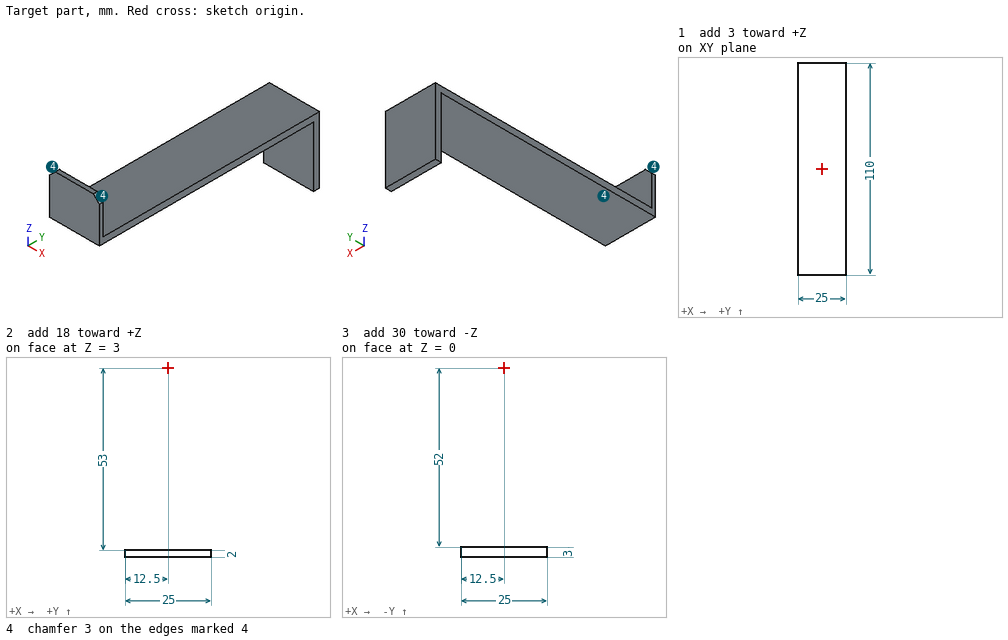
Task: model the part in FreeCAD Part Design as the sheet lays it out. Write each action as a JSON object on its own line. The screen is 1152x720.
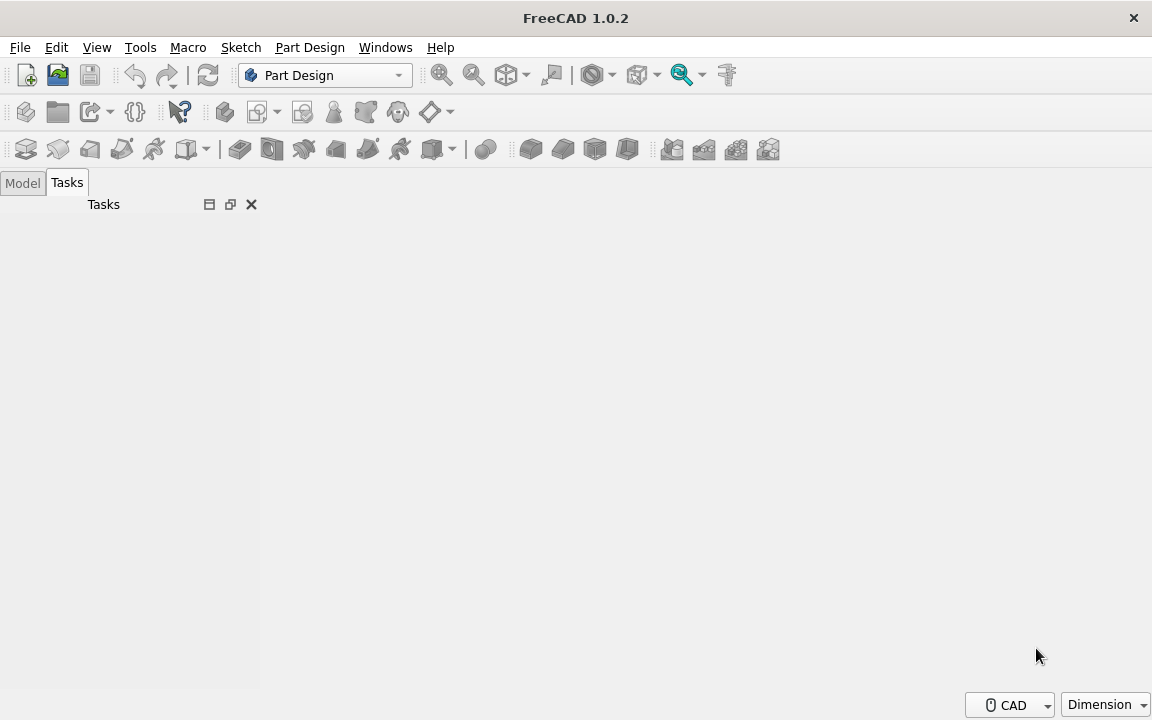
{"action": "left_click", "coordinate": [26, 76]}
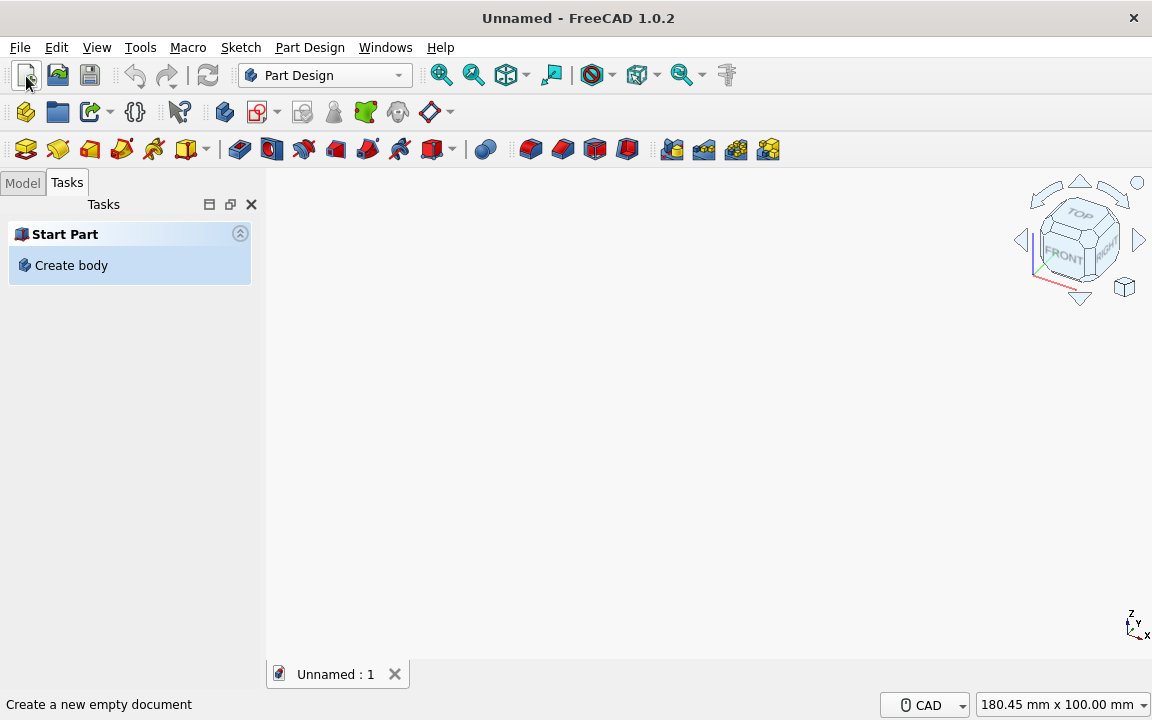
{"action": "left_click", "coordinate": [258, 112]}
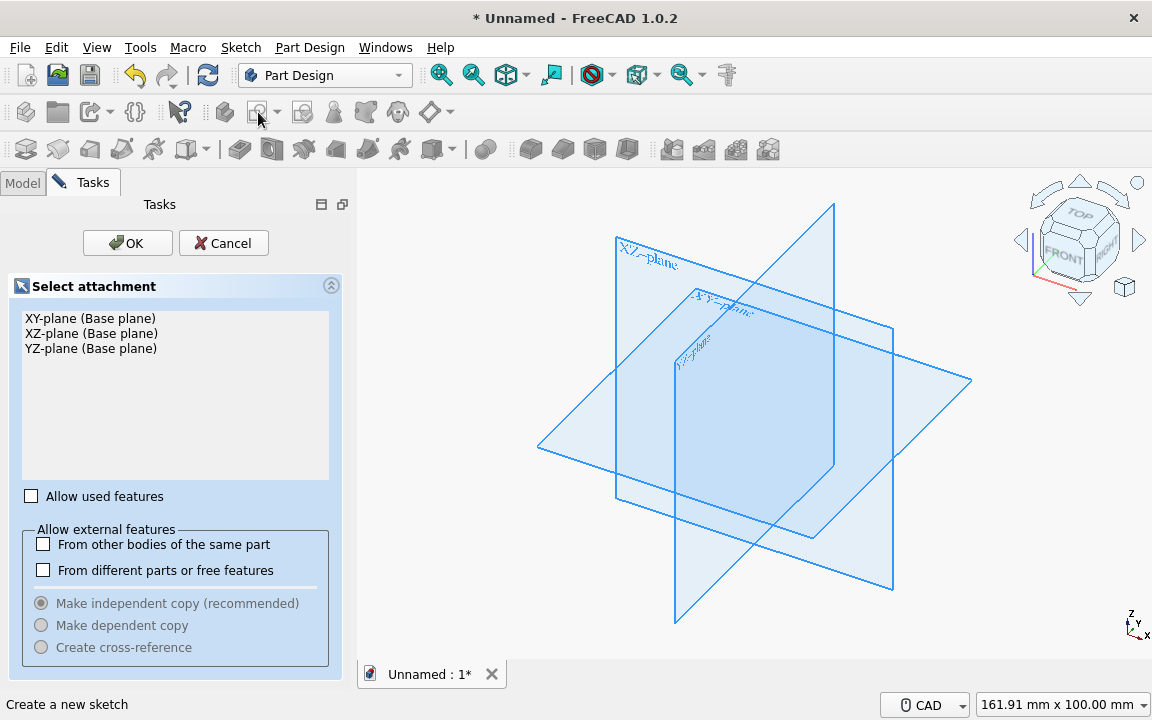
{"action": "left_click", "coordinate": [82, 318]}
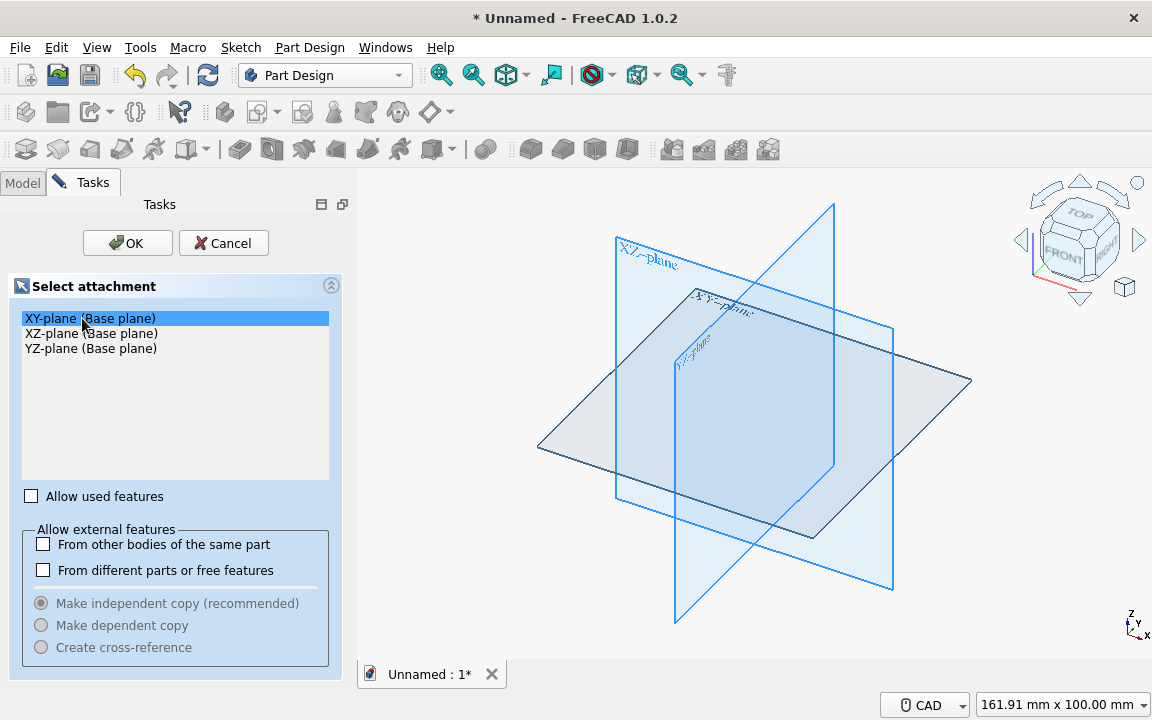
{"action": "left_click", "coordinate": [128, 243]}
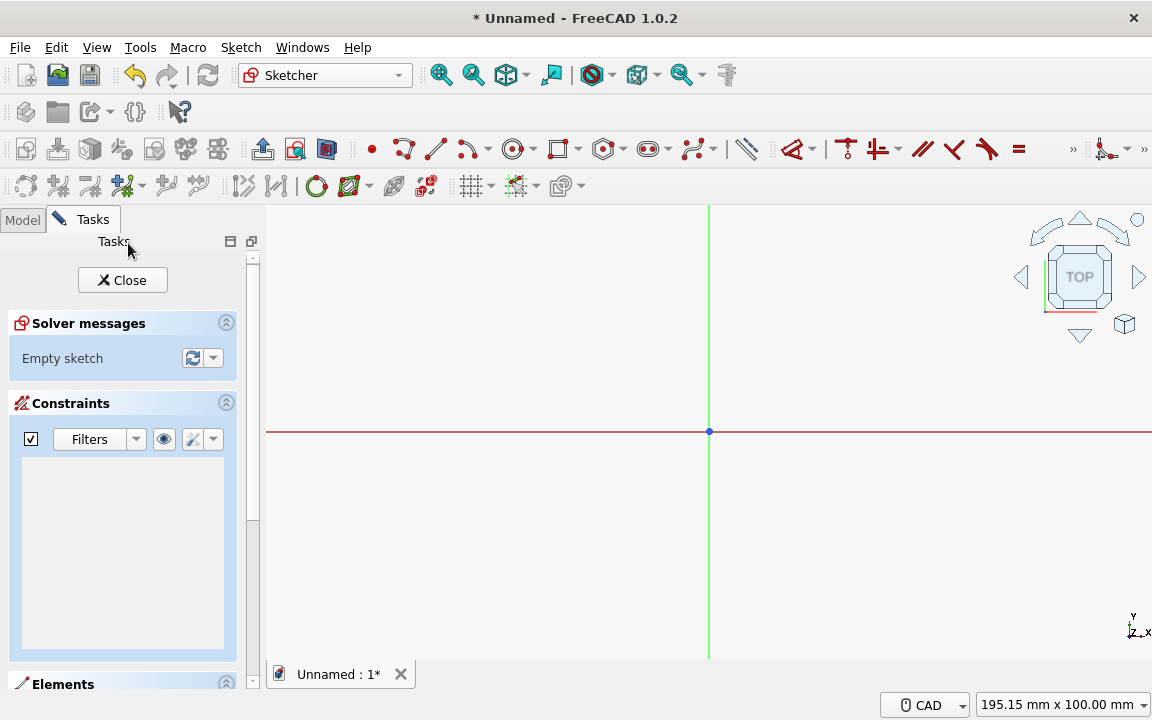
{"action": "scroll", "coordinate": [557, 432], "scroll_direction": "down", "scroll_amount": 3}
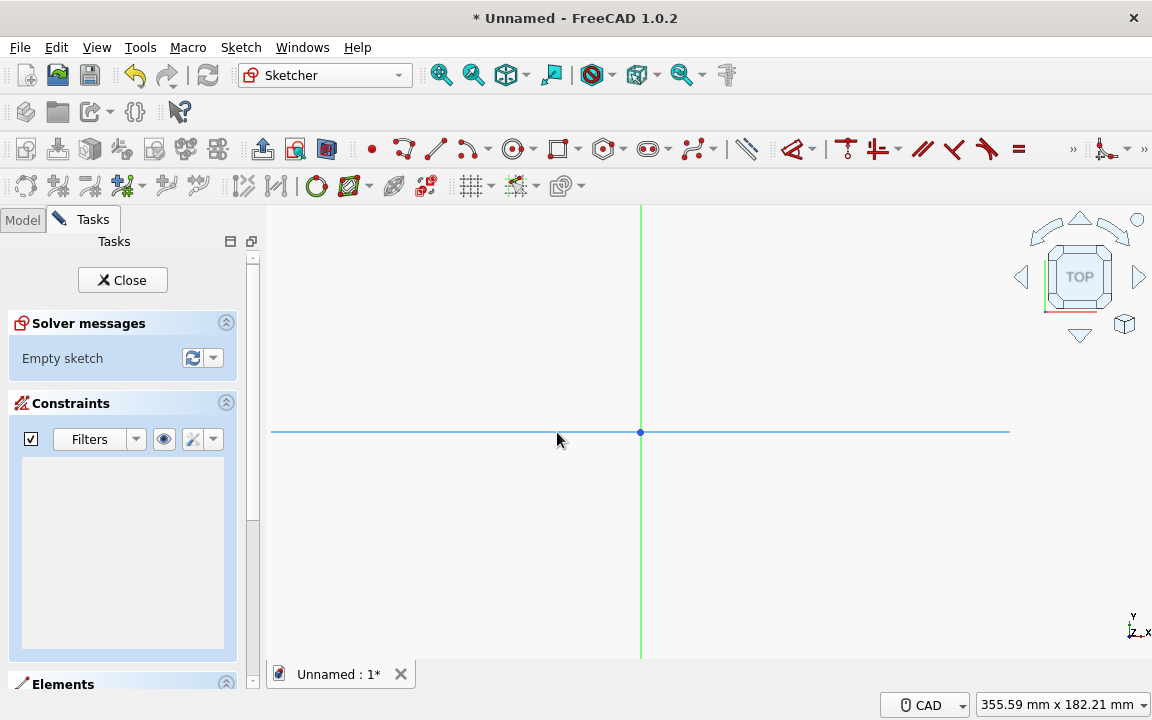
{"action": "key", "text": "g v"}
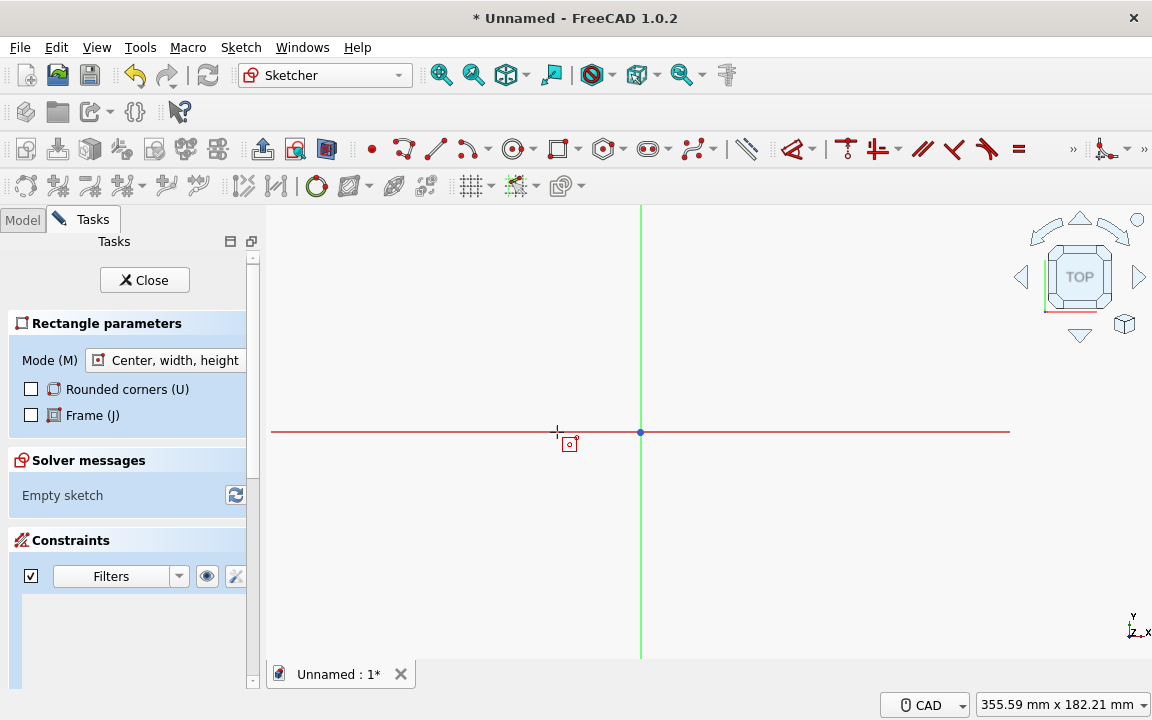
{"action": "left_click", "coordinate": [641, 432]}
{"action": "mouse_move", "coordinate": [672, 295]}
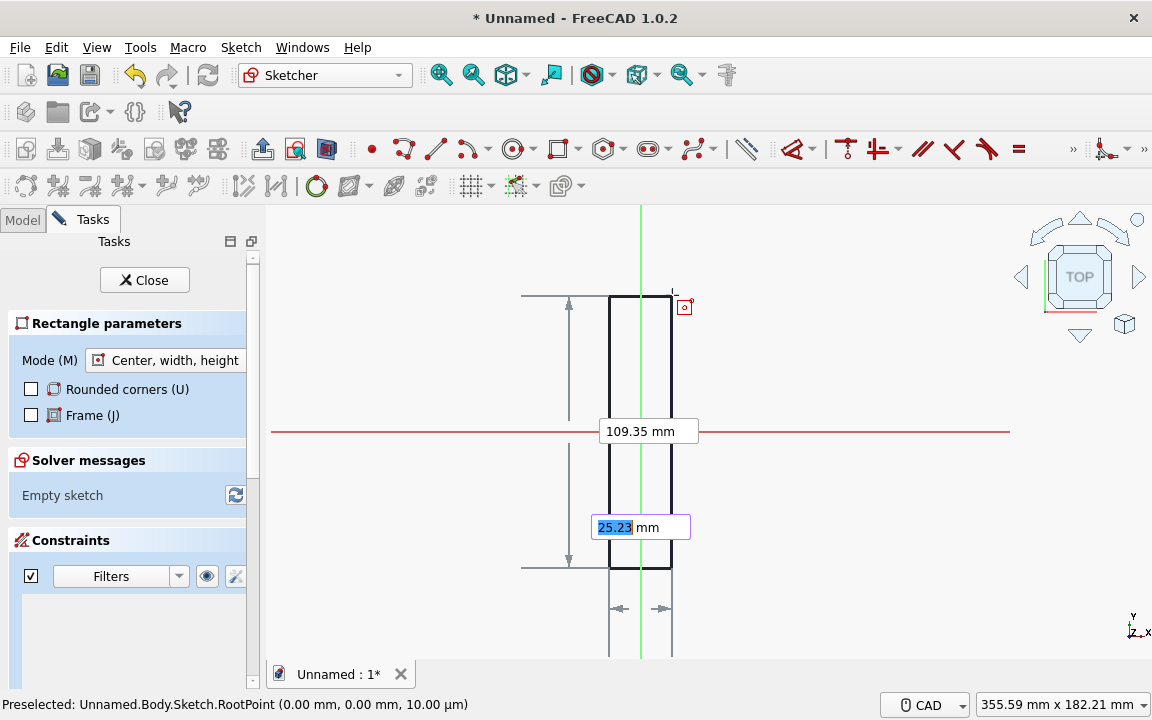
{"action": "type", "text": "25"}
{"action": "key", "text": "Tab"}
{"action": "type", "text": "110"}
{"action": "key", "text": "Return"}
{"action": "key", "text": "Escape"}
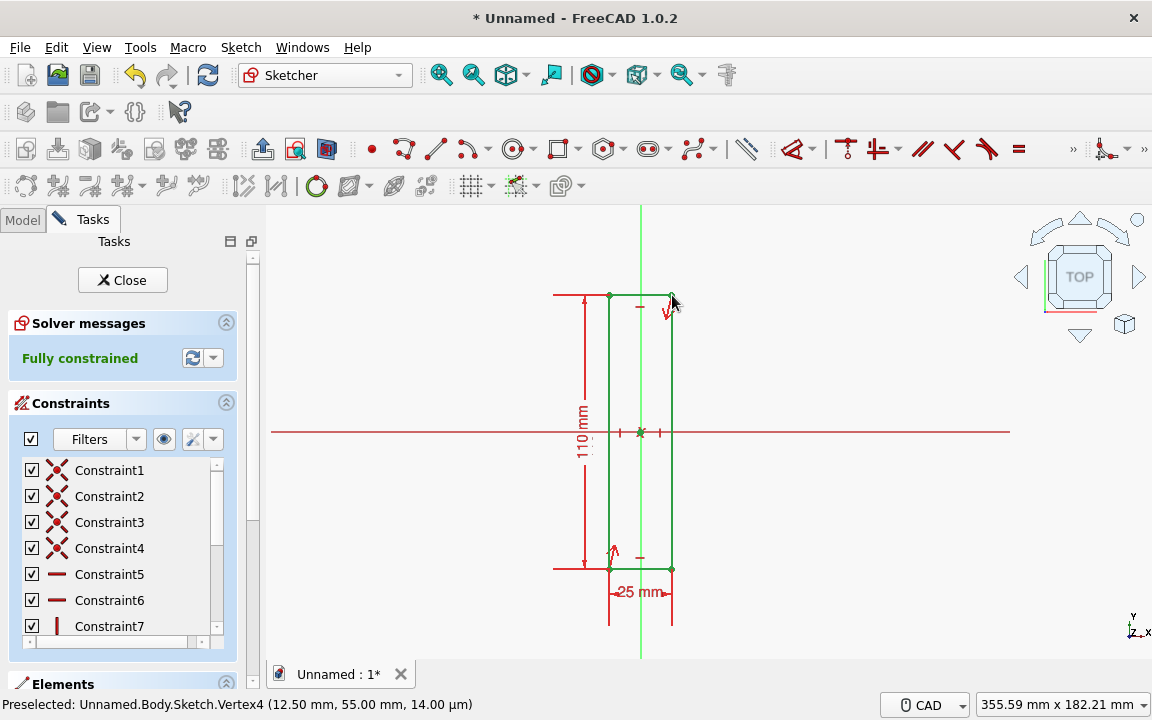
{"action": "left_click", "coordinate": [123, 280]}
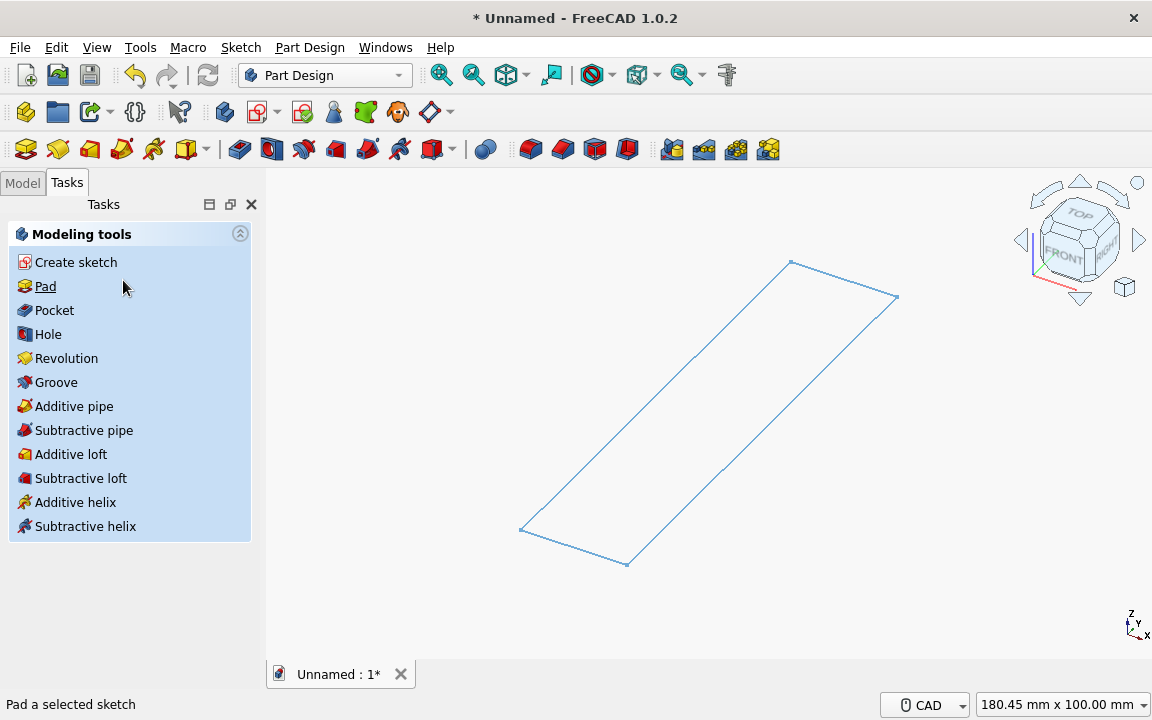
{"action": "left_click", "coordinate": [26, 150]}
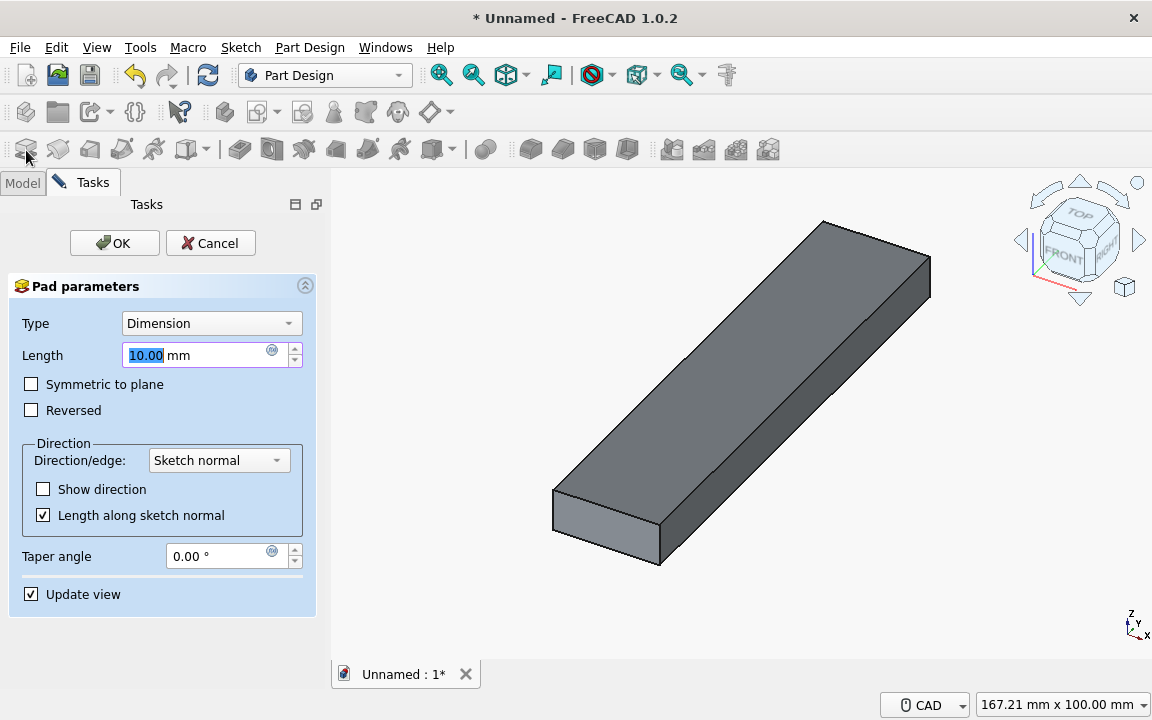
{"action": "type", "text": "3"}
{"action": "key", "text": "Tab"}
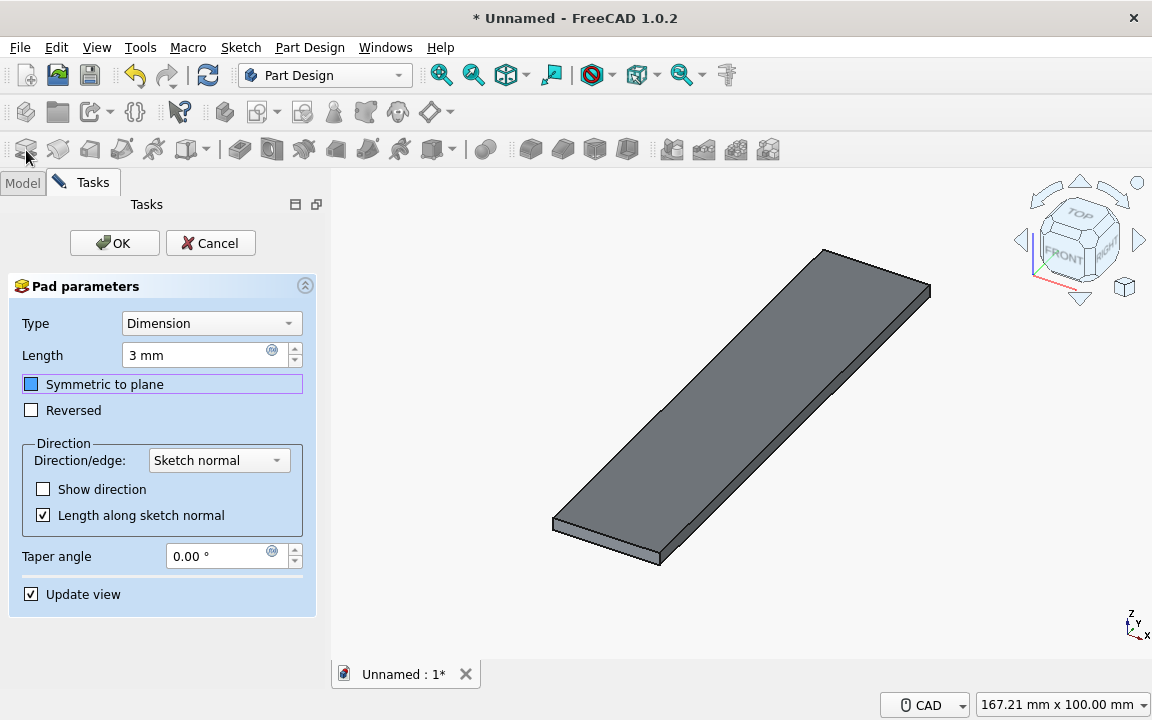
{"action": "left_click", "coordinate": [115, 243]}